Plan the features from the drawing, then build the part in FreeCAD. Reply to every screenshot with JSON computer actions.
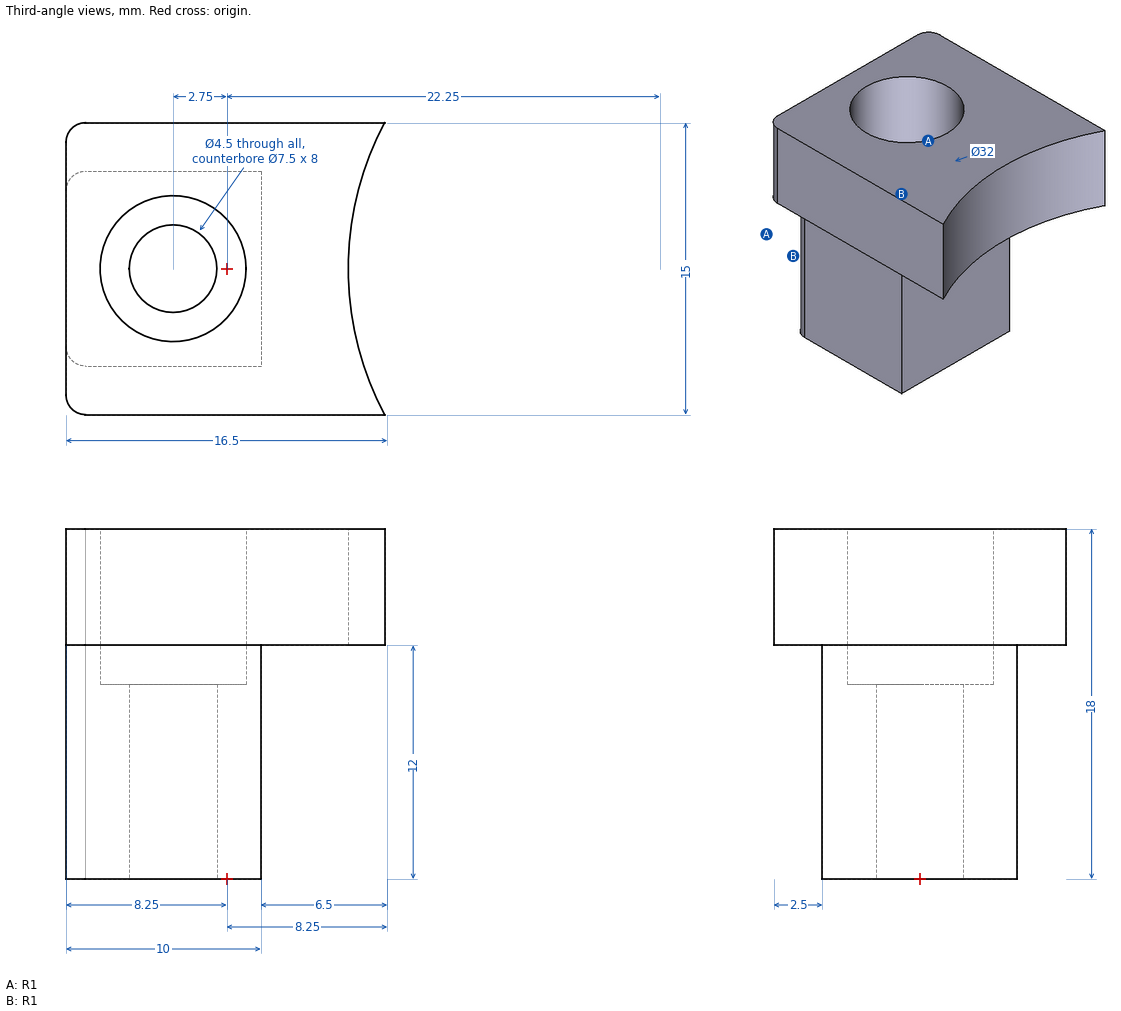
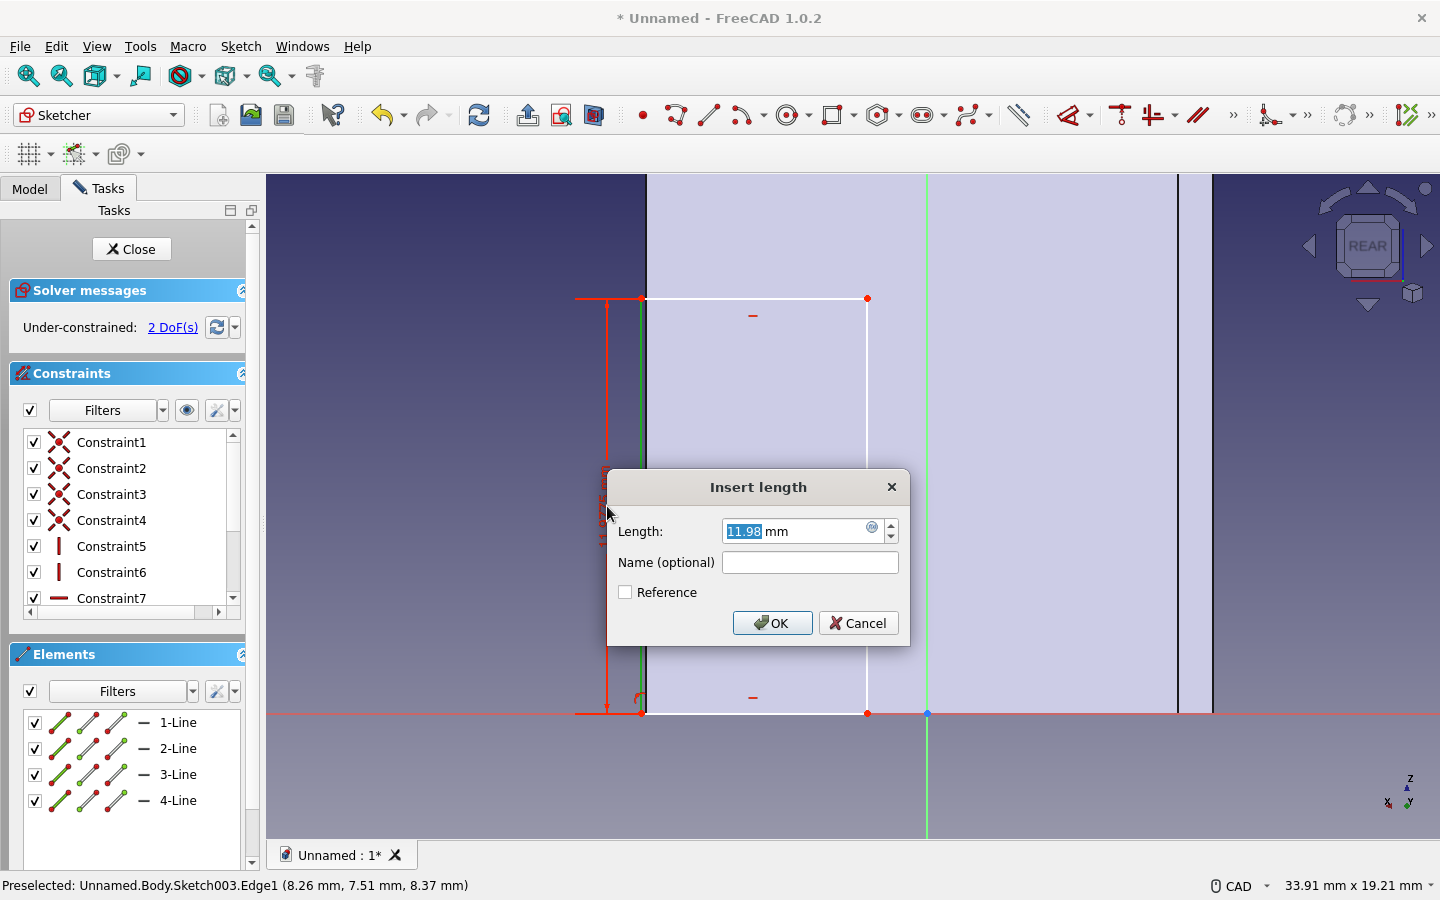
{"action": "type", "text": "12"}
{"action": "key", "text": "Return"}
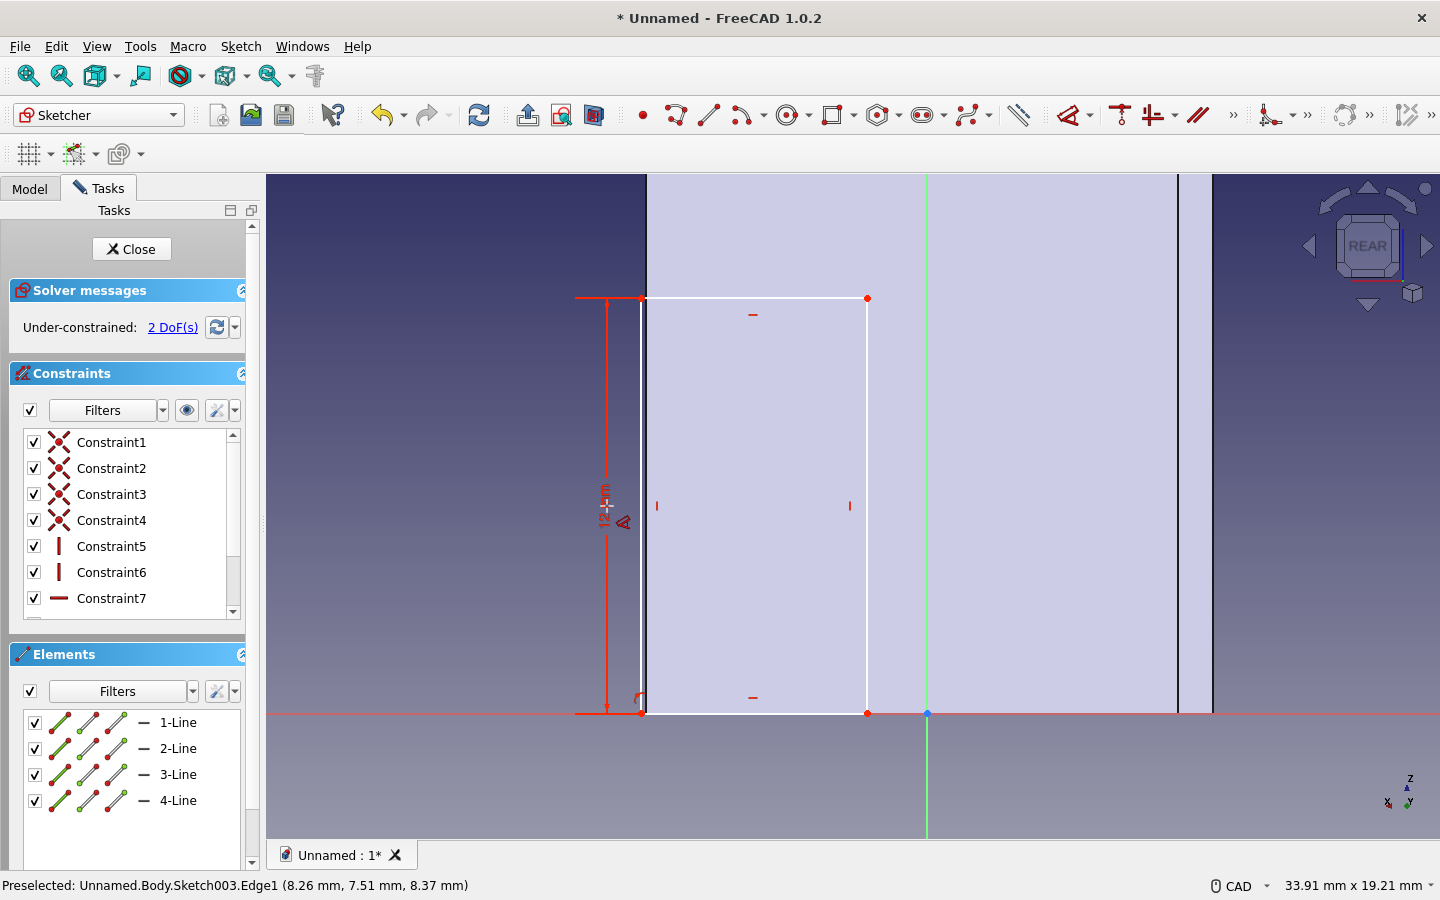
{"action": "left_click", "coordinate": [709, 714]}
{"action": "left_click", "coordinate": [754, 748]}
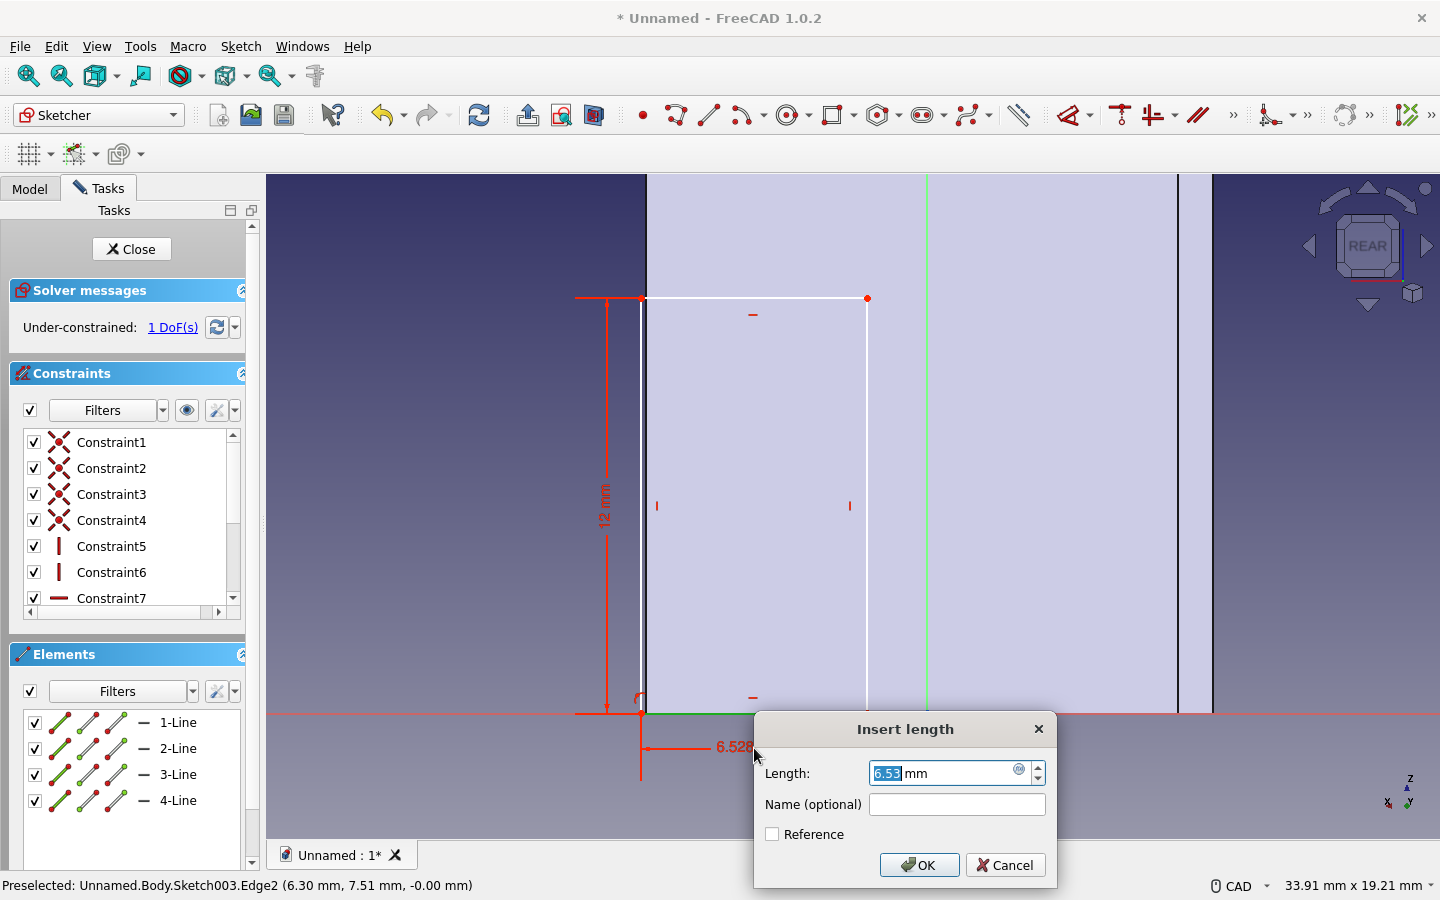
{"action": "type", "text": "6.5"}
{"action": "key", "text": "Return"}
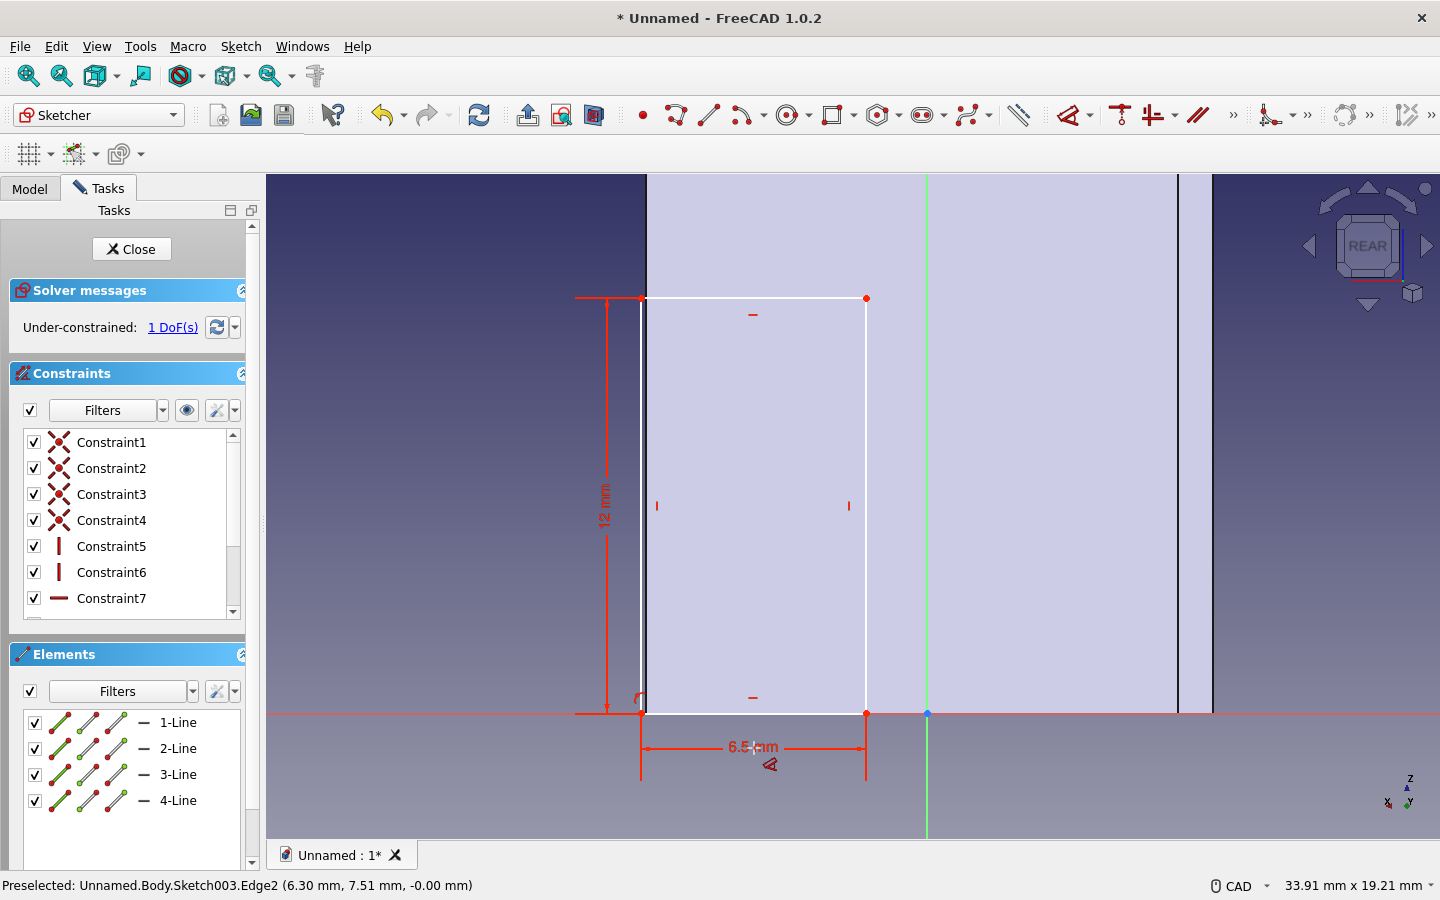
{"action": "left_click", "coordinate": [641, 298]}
{"action": "left_click", "coordinate": [850, 748]}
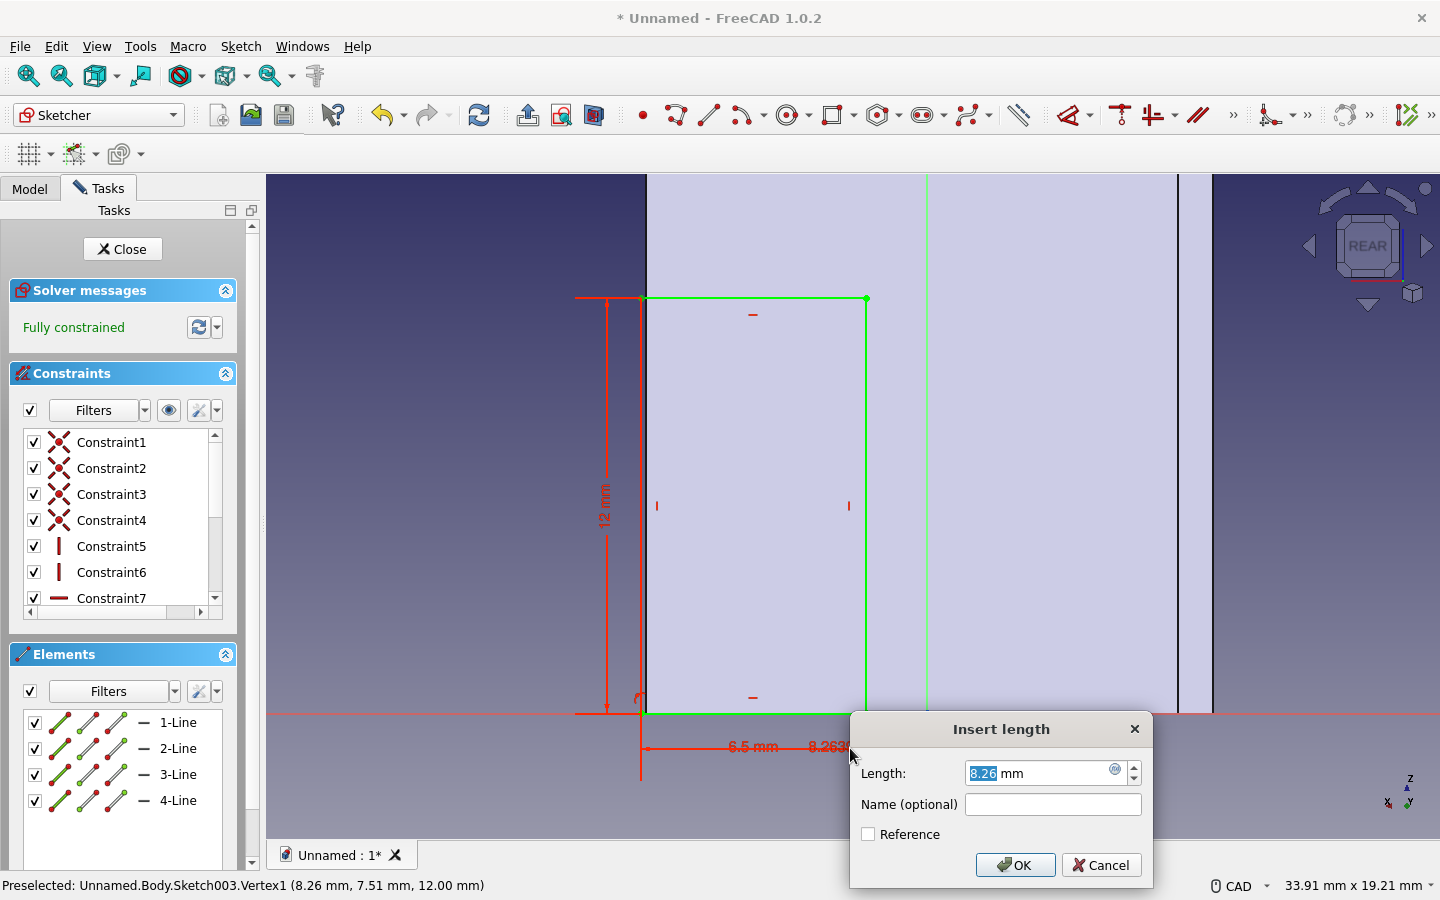
{"action": "type", "text": "8.25"}
{"action": "key", "text": "Return"}
{"action": "key", "text": "Escape"}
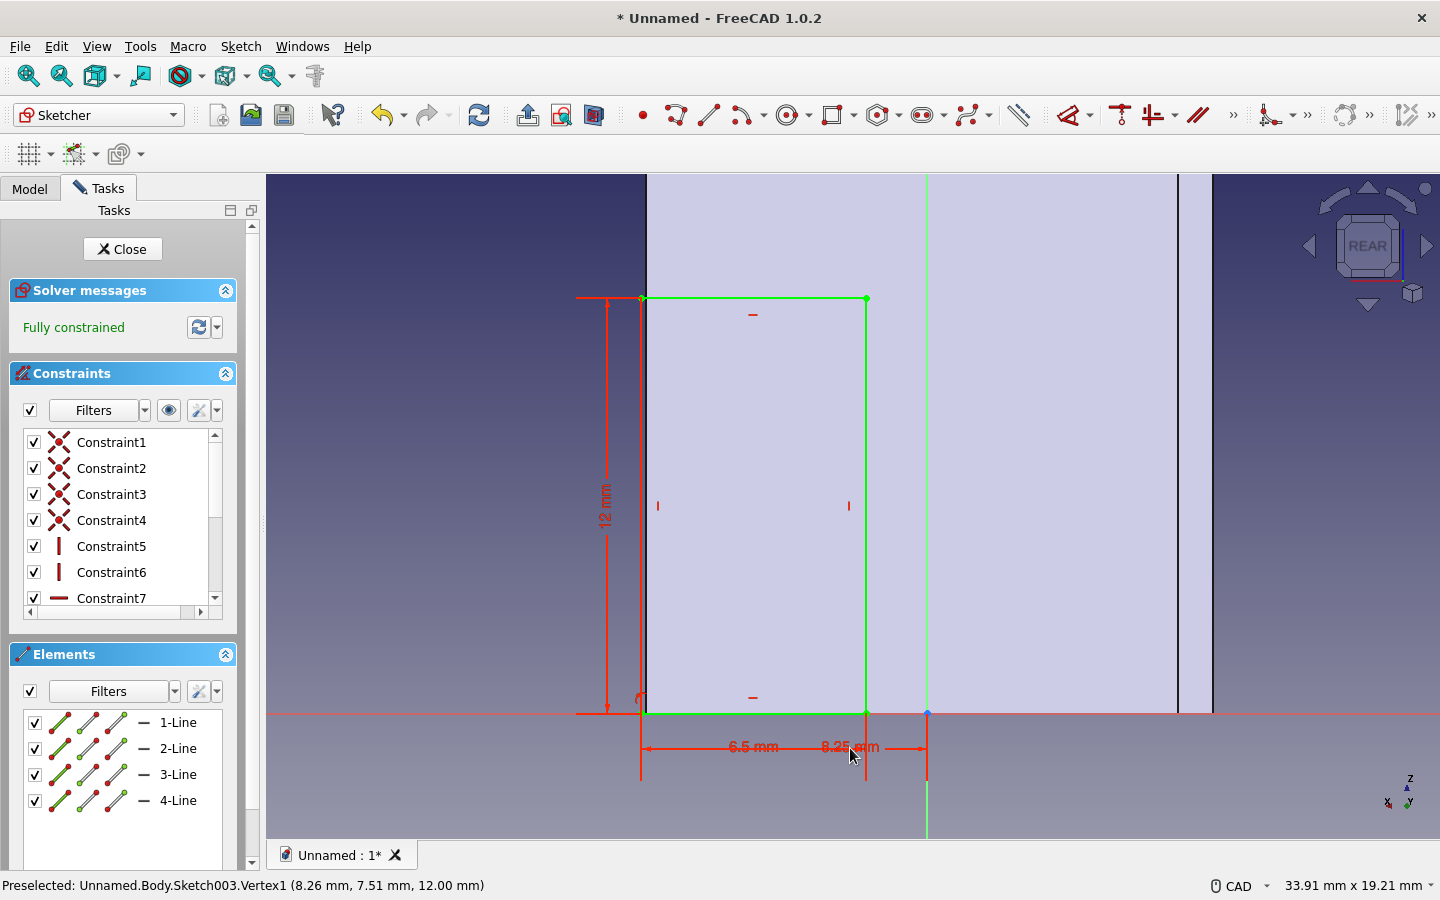
{"action": "left_click", "coordinate": [123, 249]}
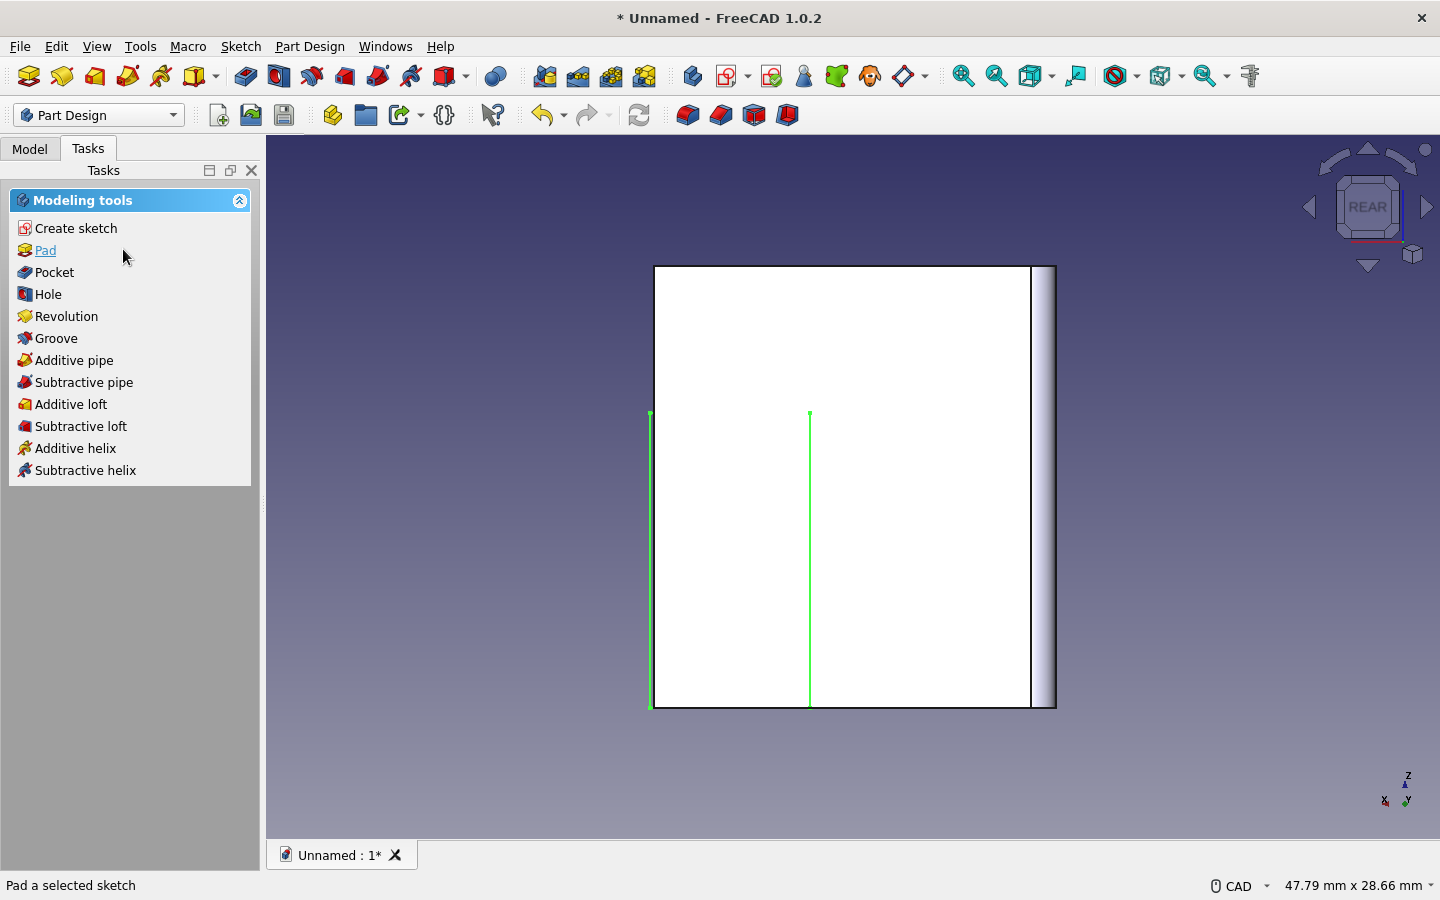
{"action": "left_click", "coordinate": [246, 76]}